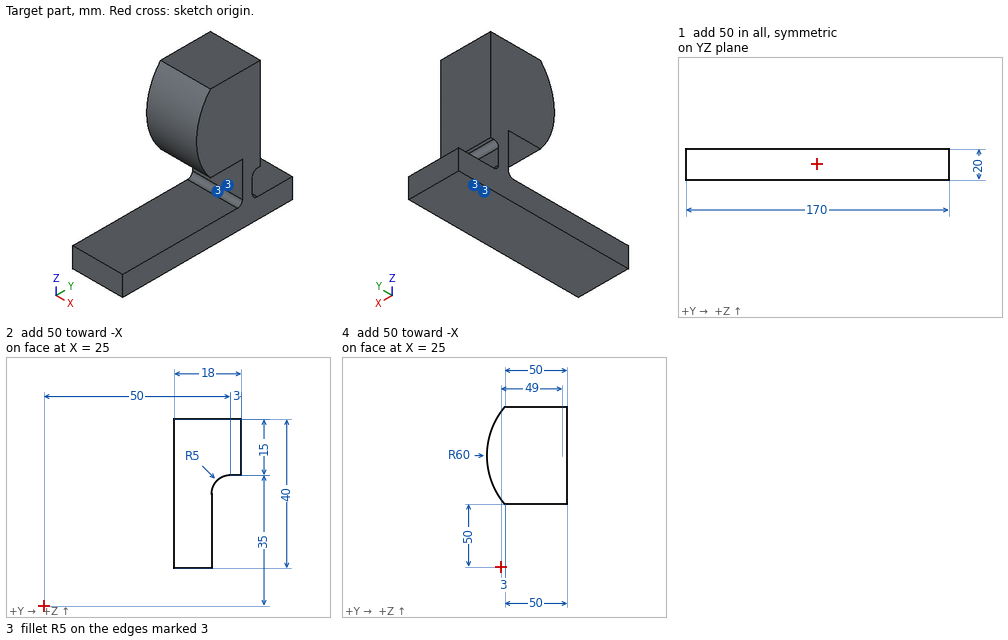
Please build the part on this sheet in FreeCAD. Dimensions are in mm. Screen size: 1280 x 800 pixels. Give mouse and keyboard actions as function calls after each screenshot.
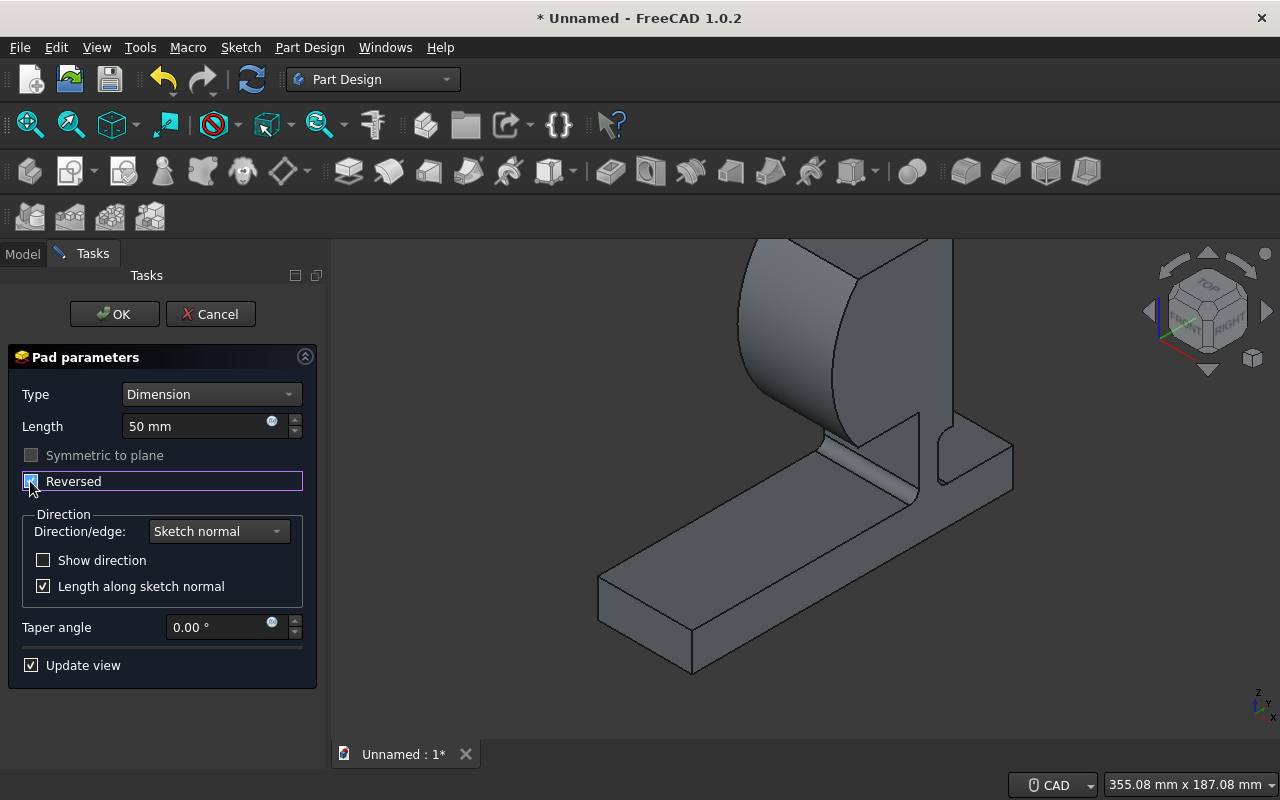
click(115, 314)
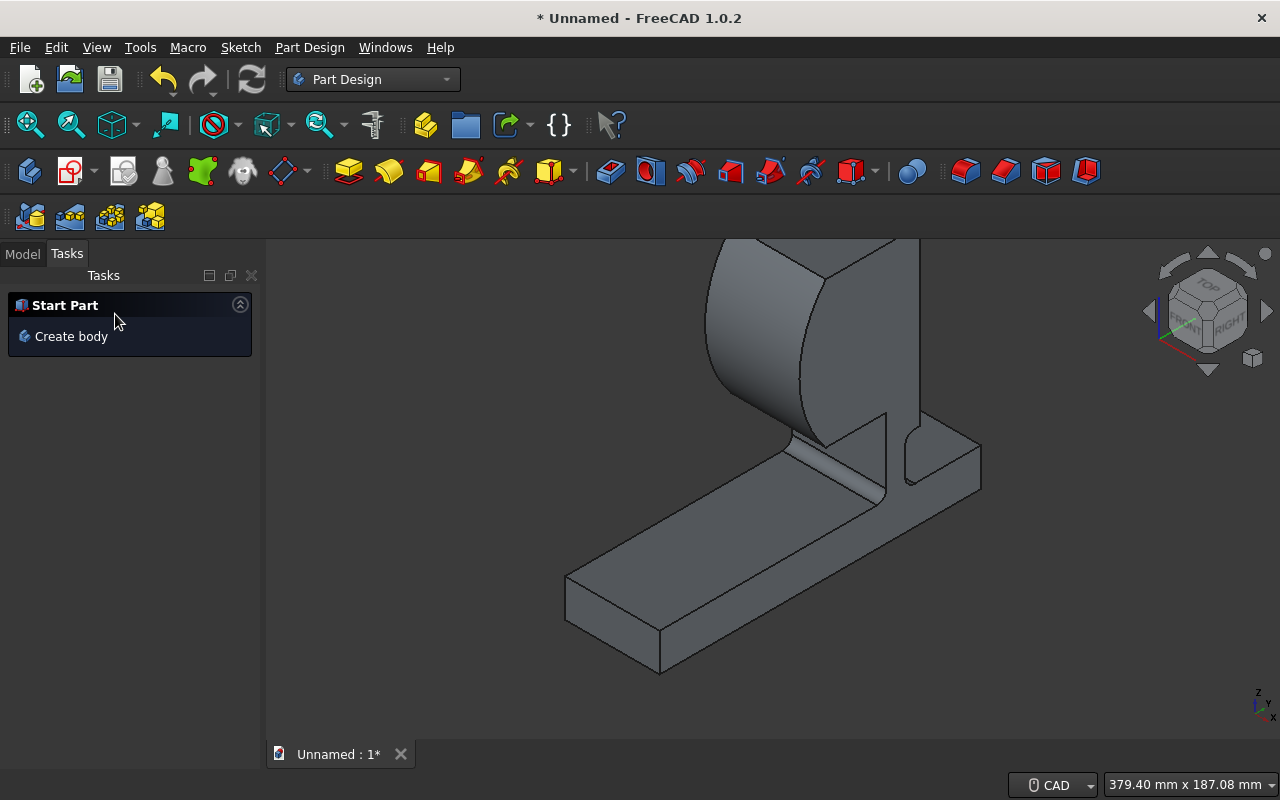
click(32, 126)